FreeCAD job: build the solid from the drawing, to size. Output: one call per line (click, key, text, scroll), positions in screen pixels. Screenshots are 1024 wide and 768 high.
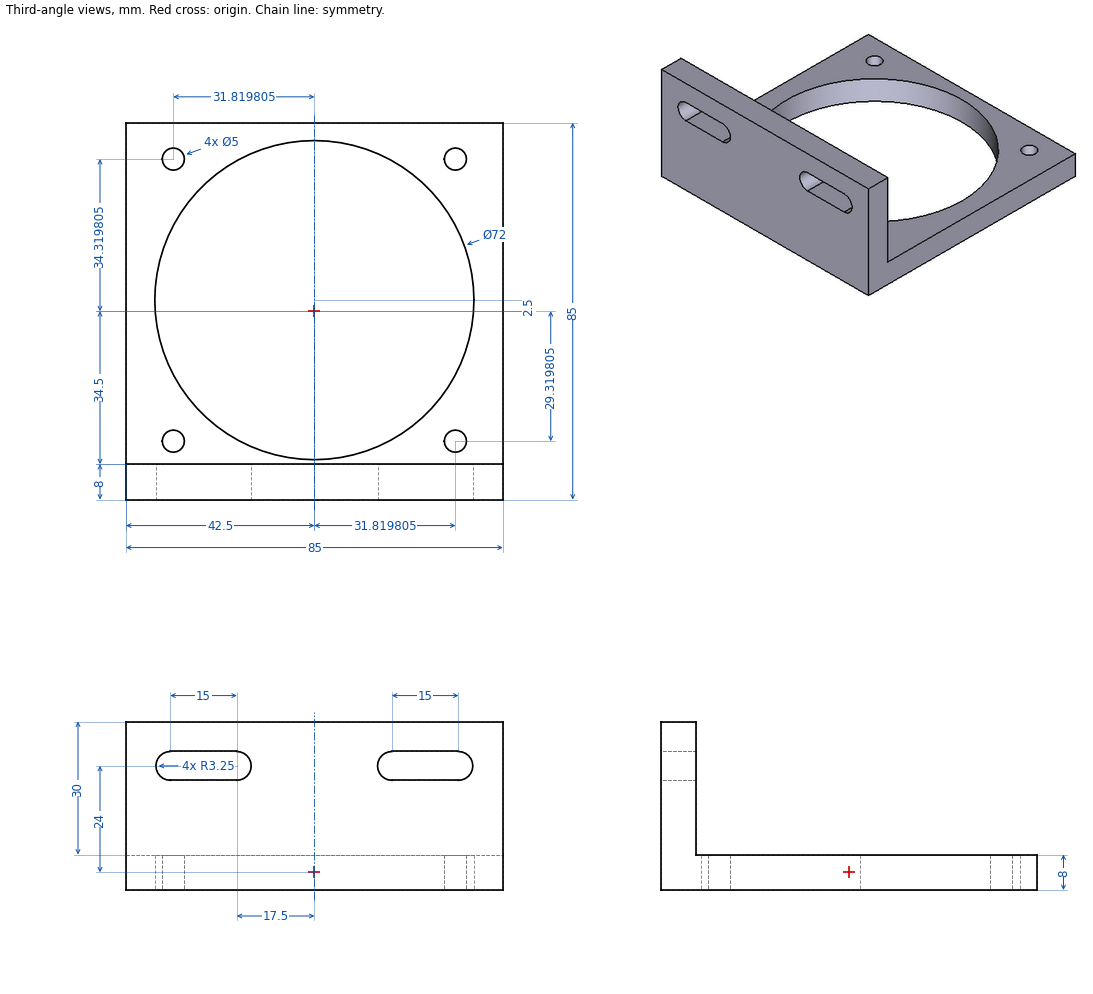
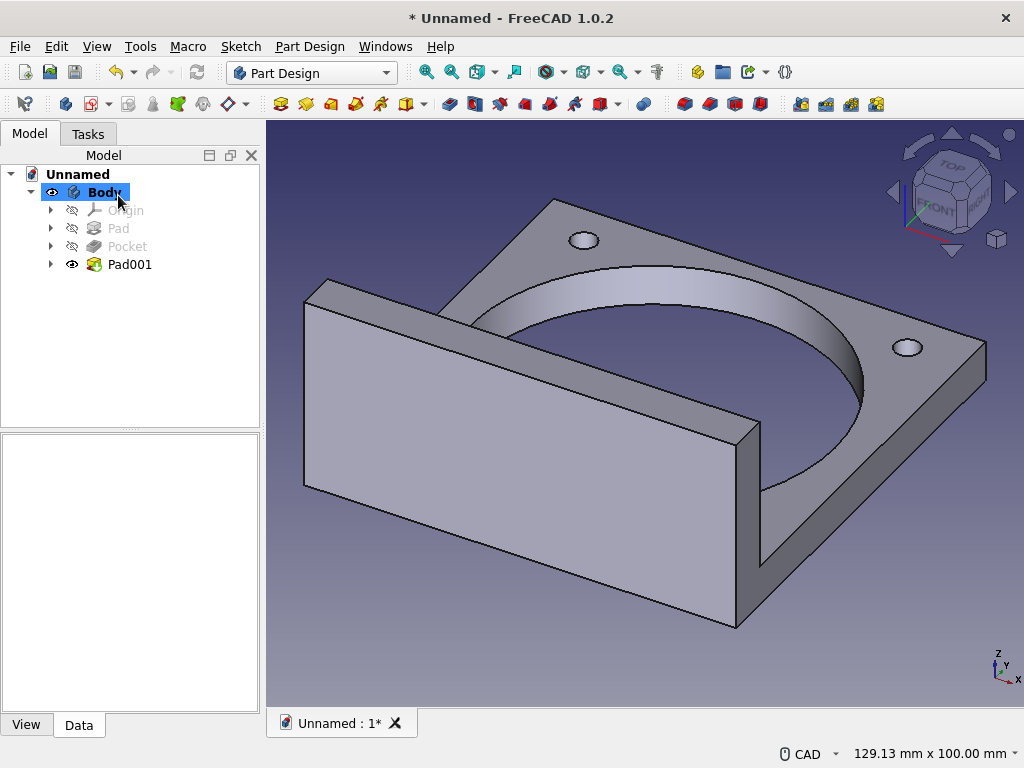
click(427, 72)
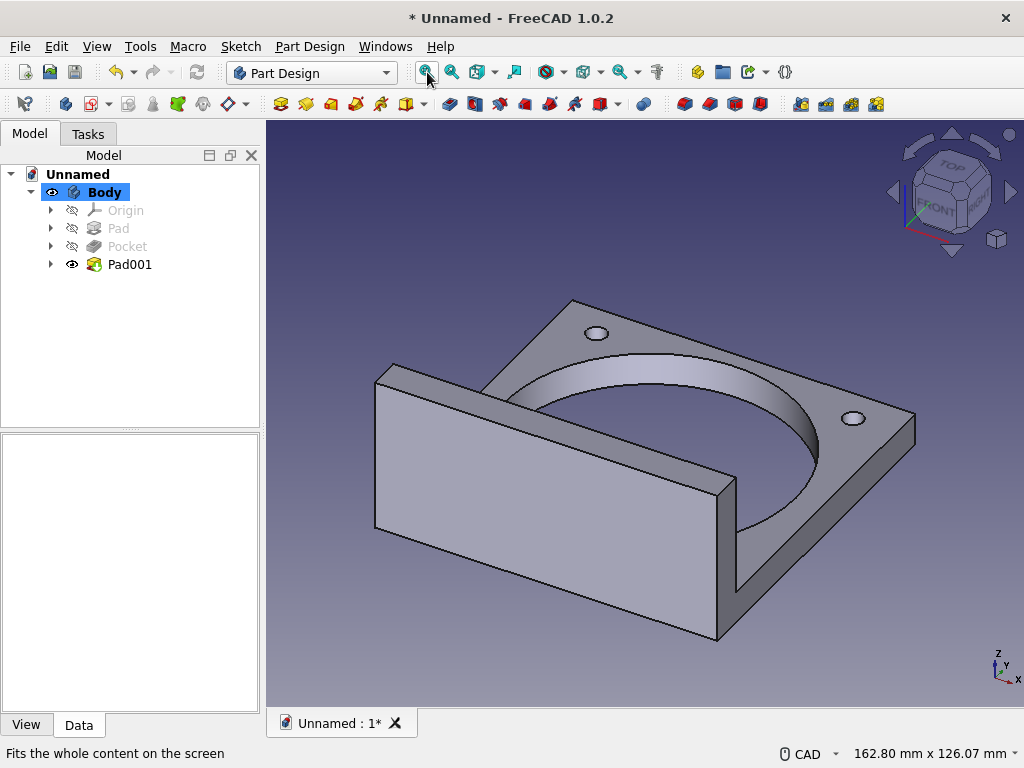
key(4)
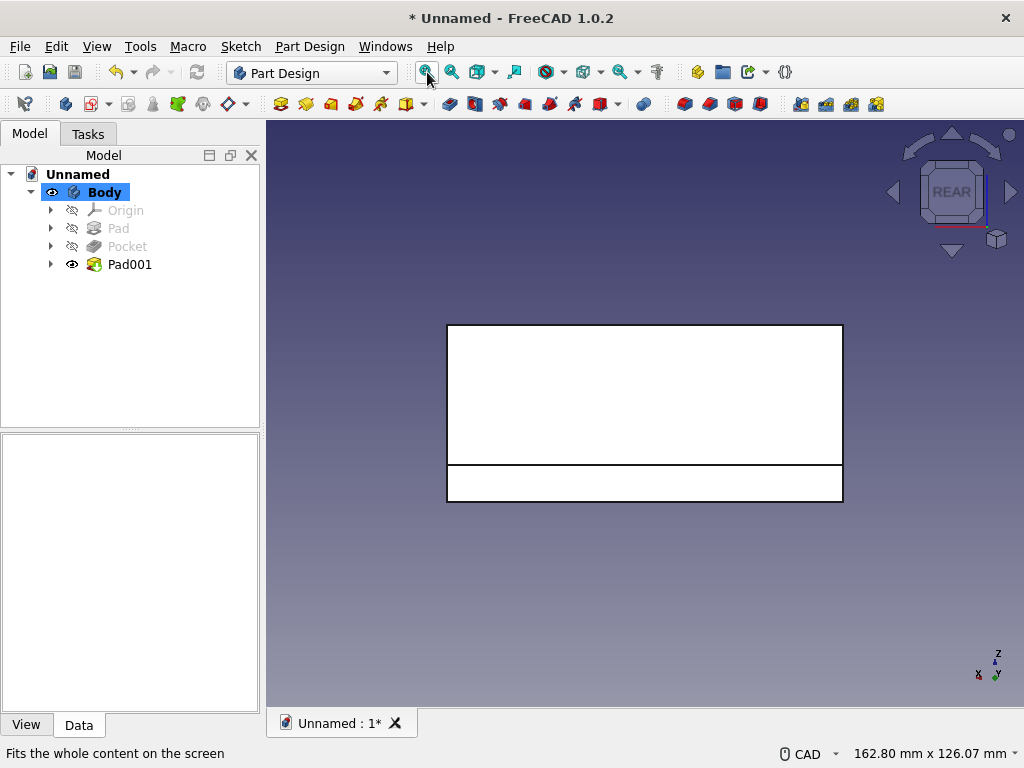
click(532, 394)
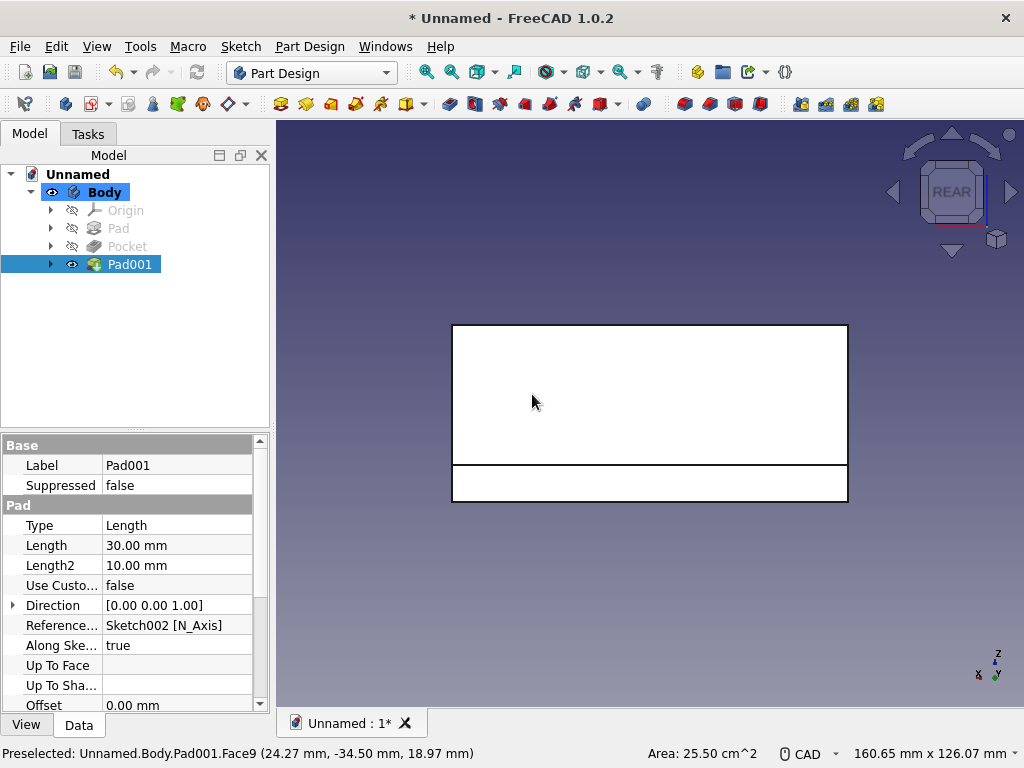
click(90, 104)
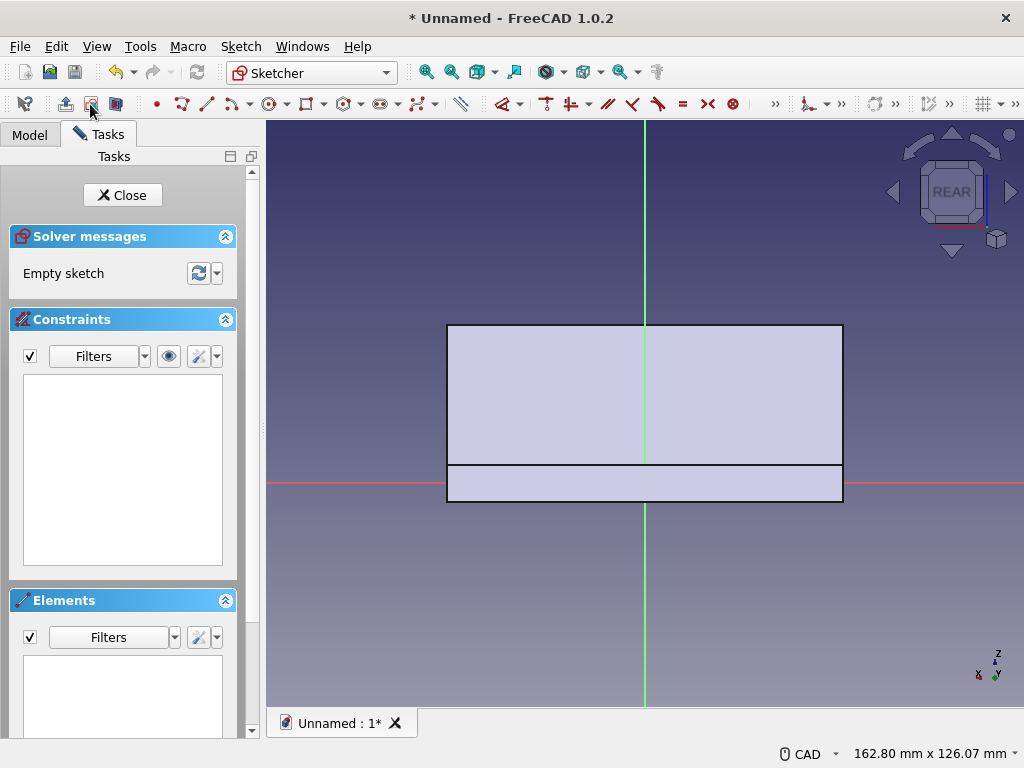
click(380, 104)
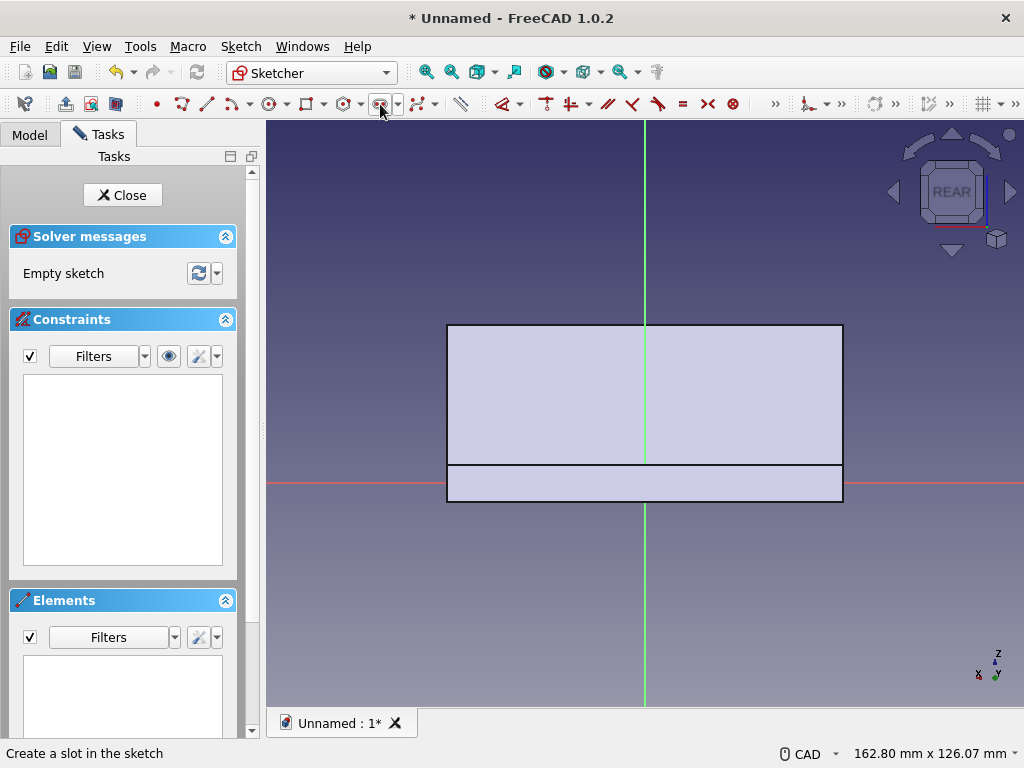
scroll(726, 372, up, 3)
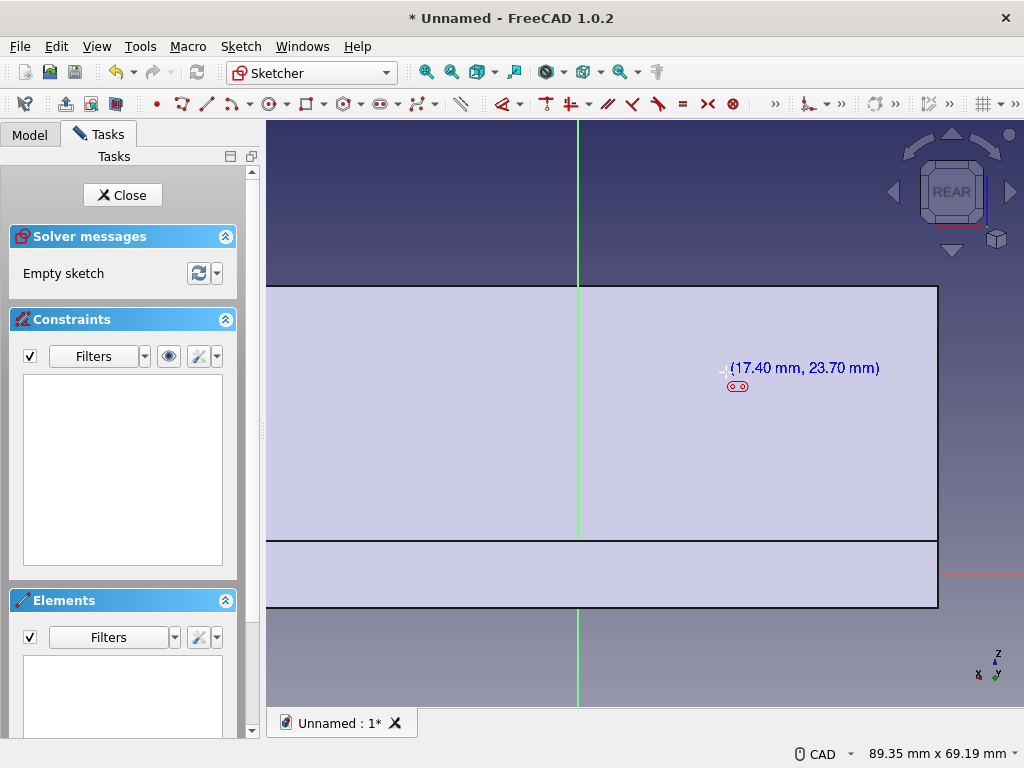
click(726, 371)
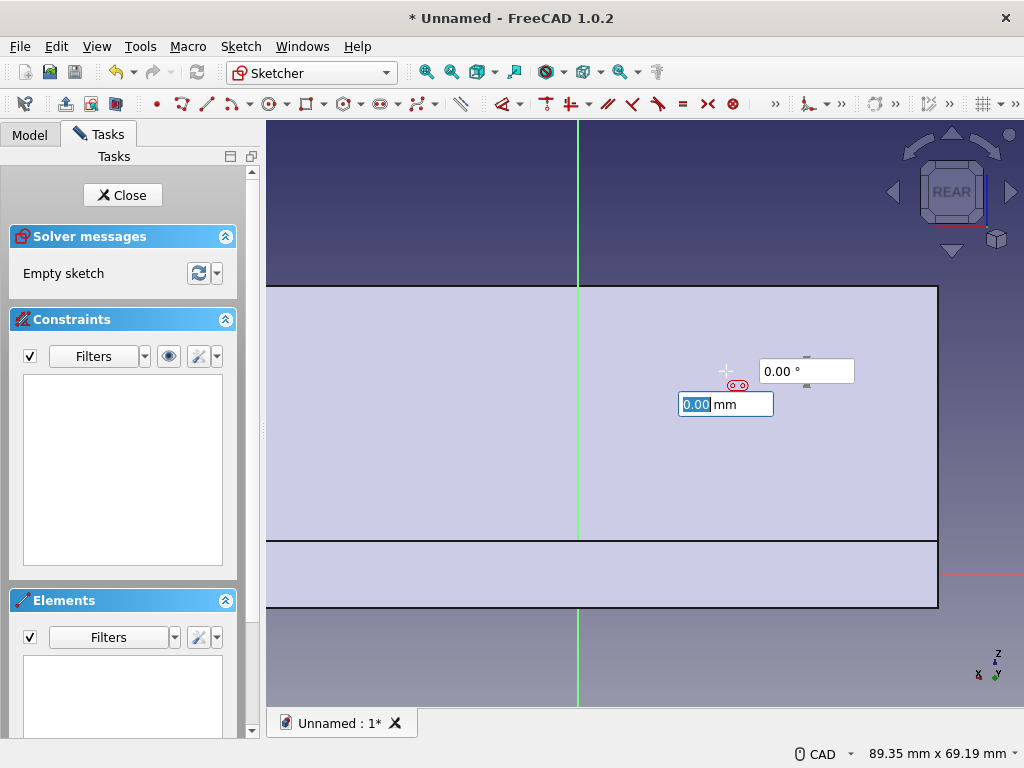
click(854, 371)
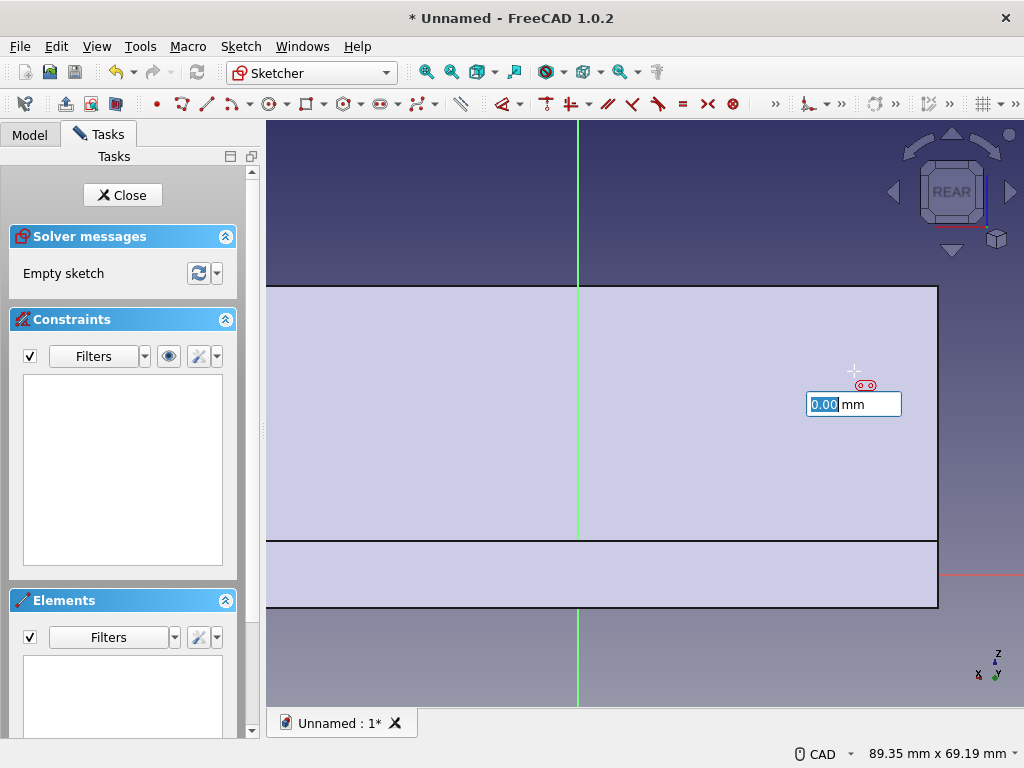
click(790, 398)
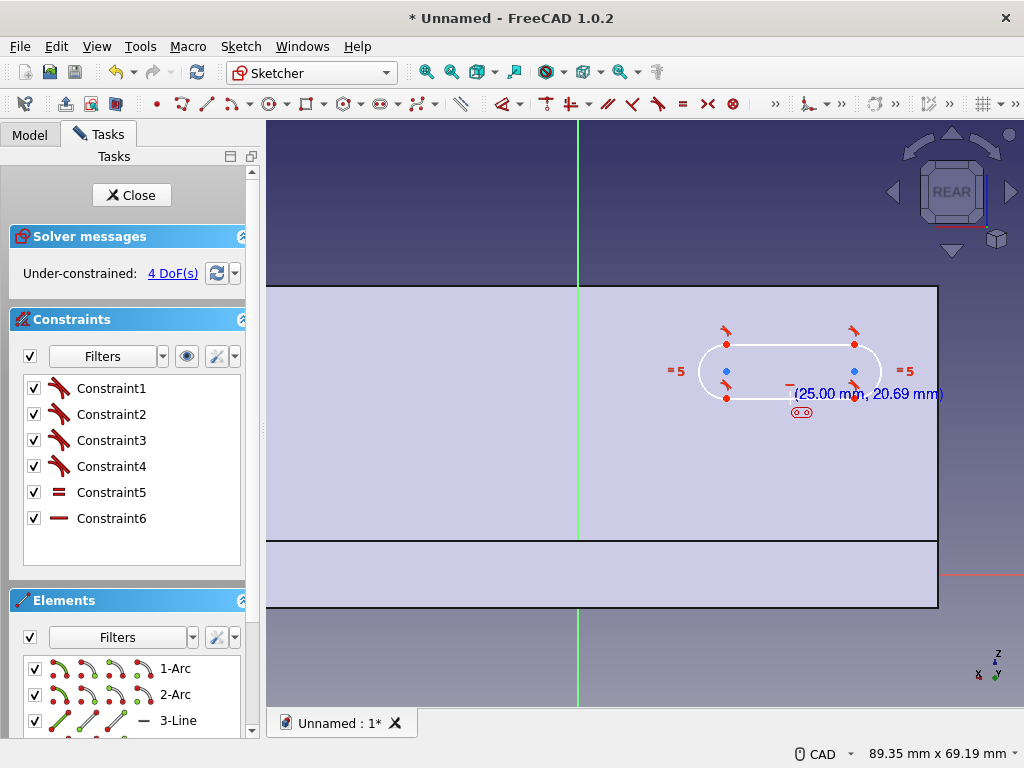
click(302, 371)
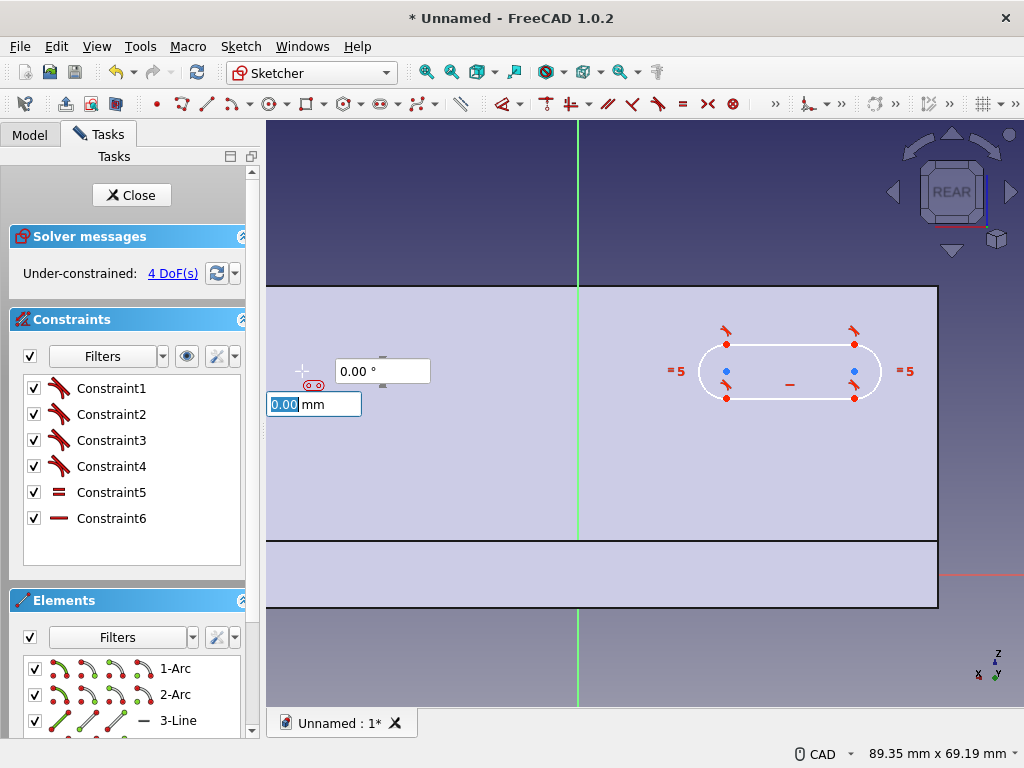
click(429, 371)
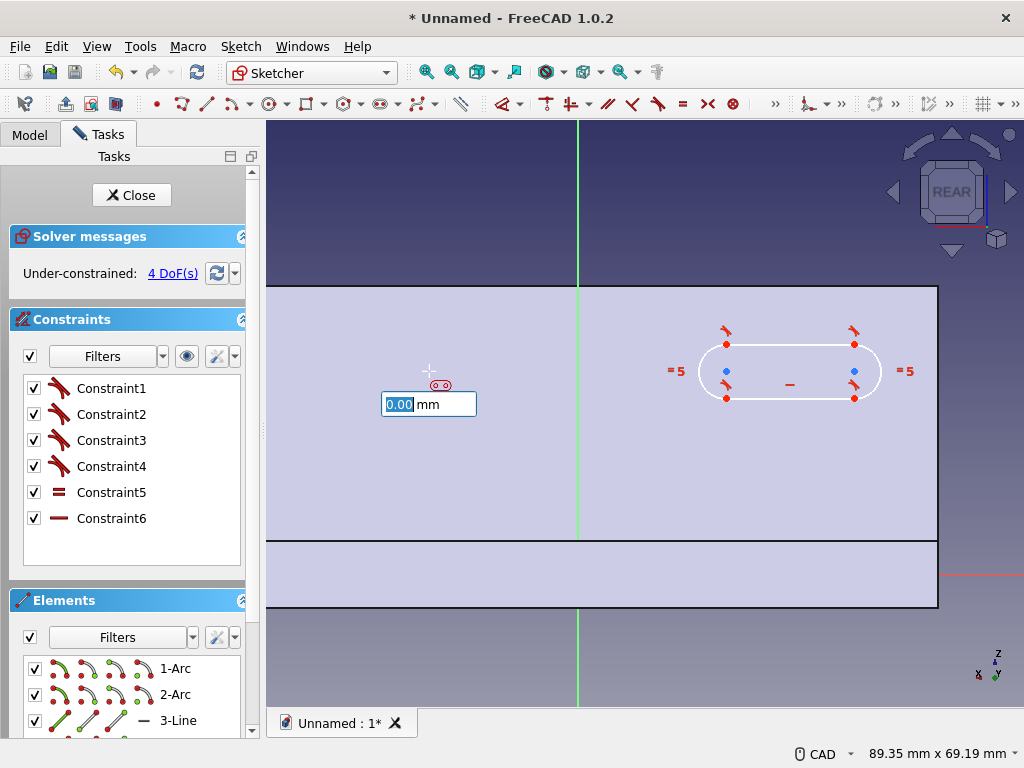
click(366, 398)
key(Escape)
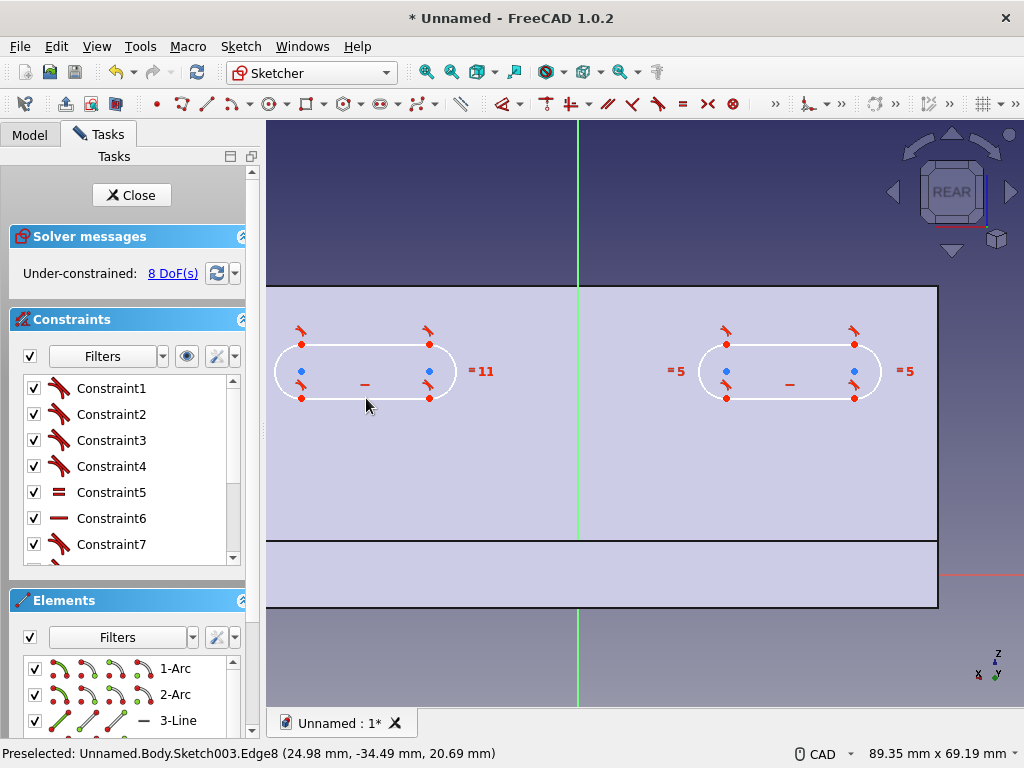
click(704, 356)